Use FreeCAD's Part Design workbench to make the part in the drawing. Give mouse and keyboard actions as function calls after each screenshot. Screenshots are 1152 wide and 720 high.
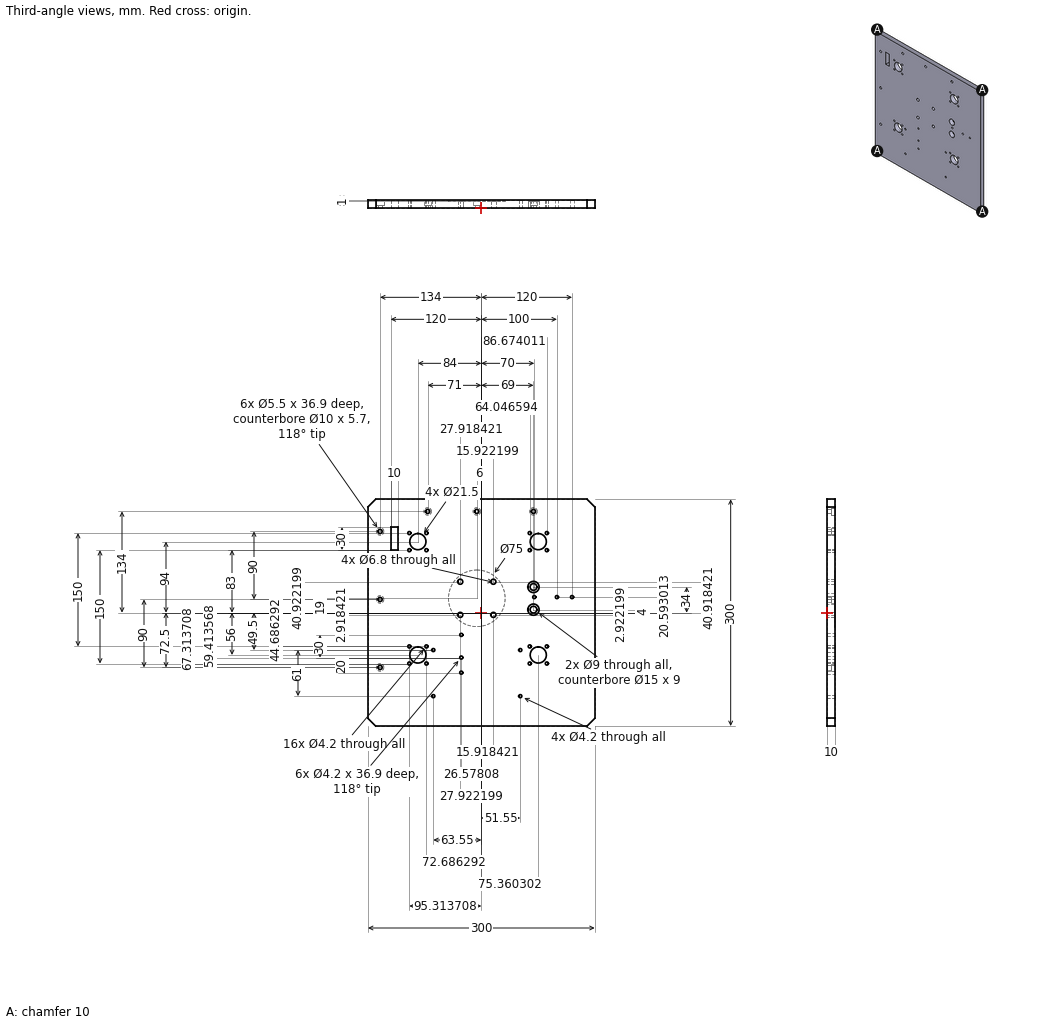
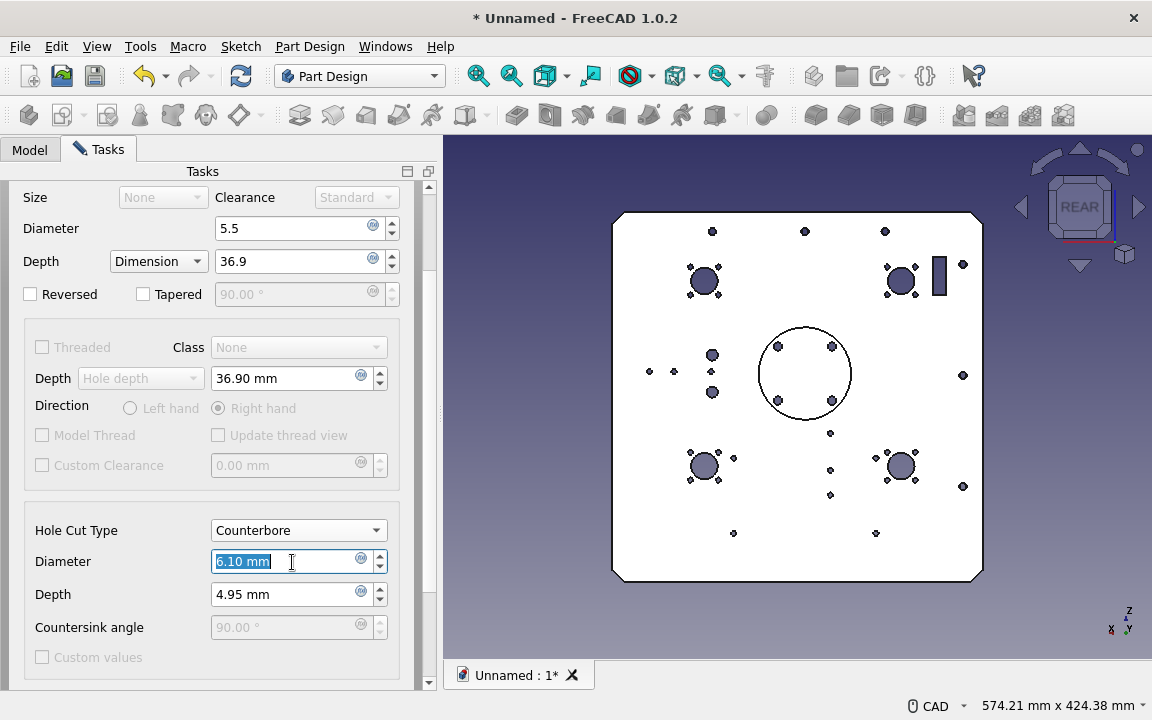
text(10)
key(Tab)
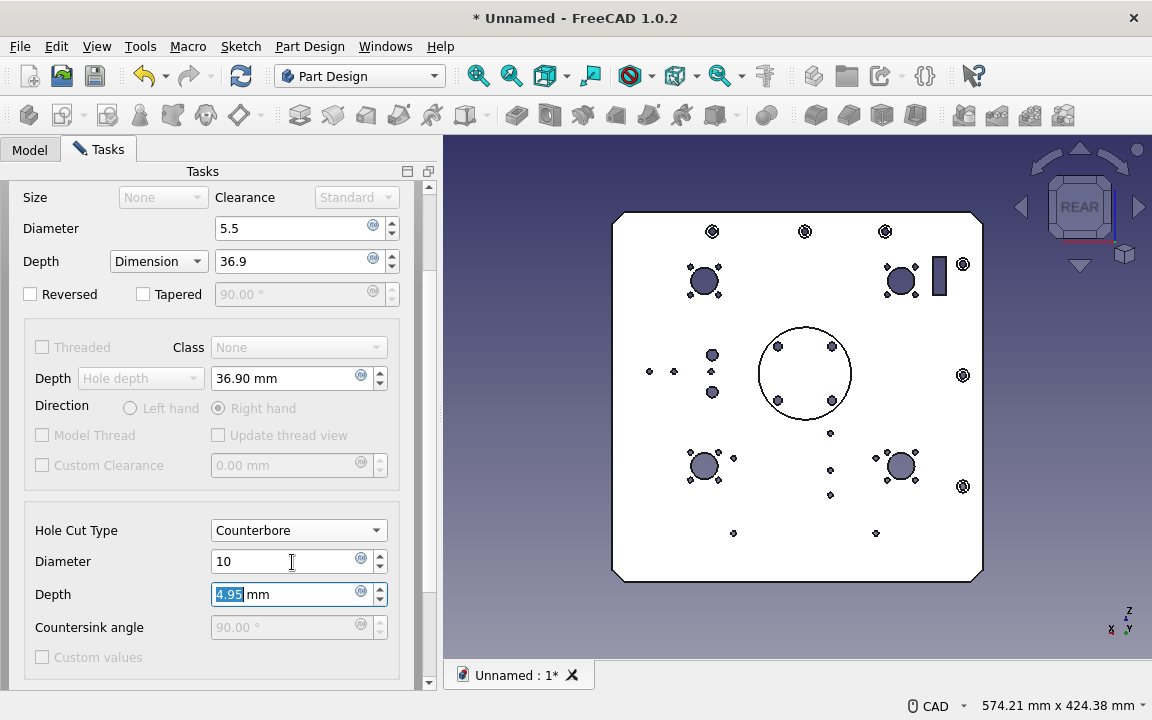
text(5.7)
key(Tab)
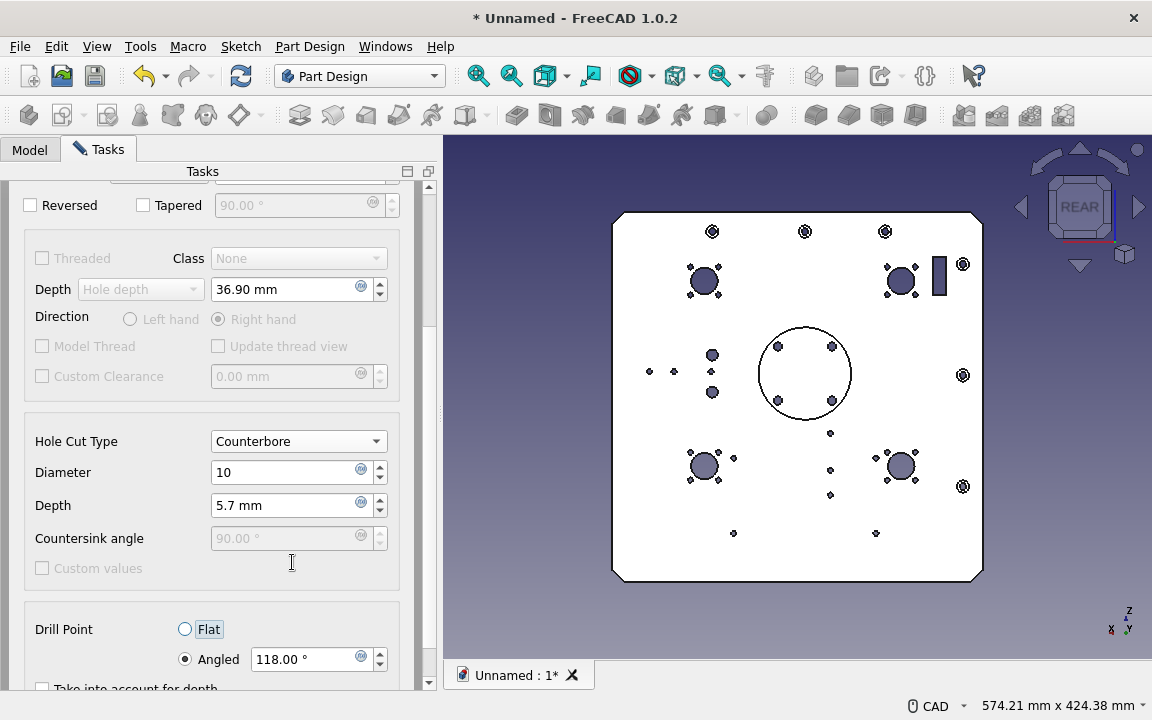
scroll(429, 436, up, 5)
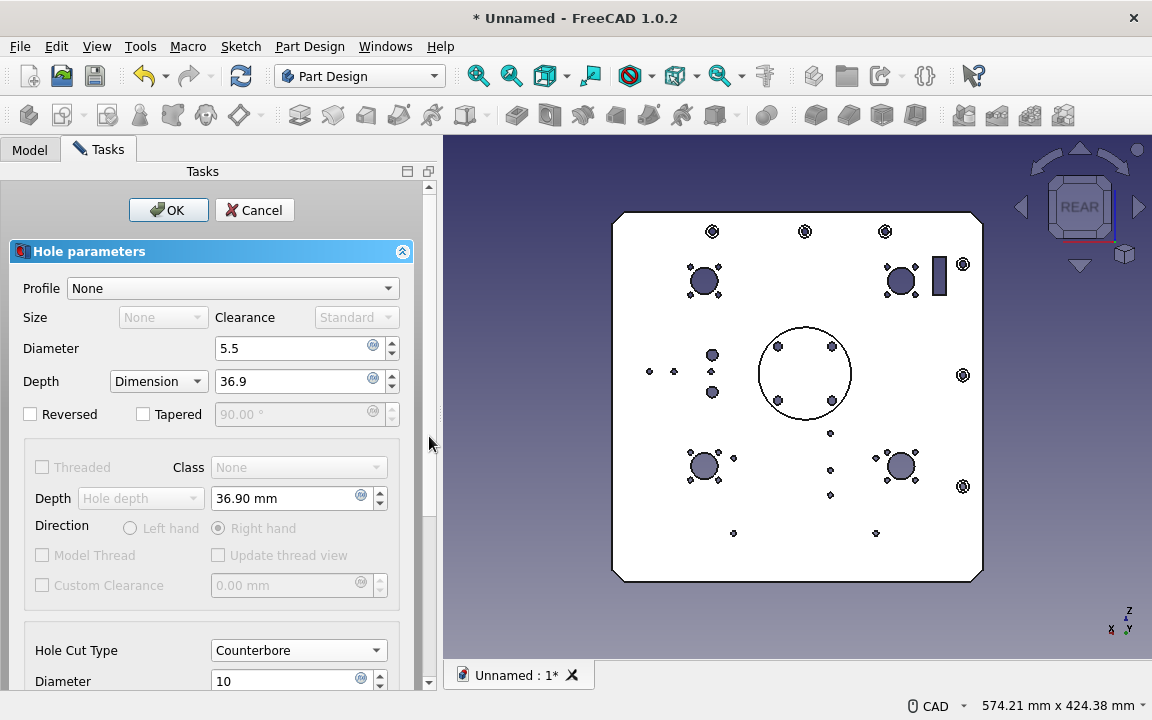
click(169, 210)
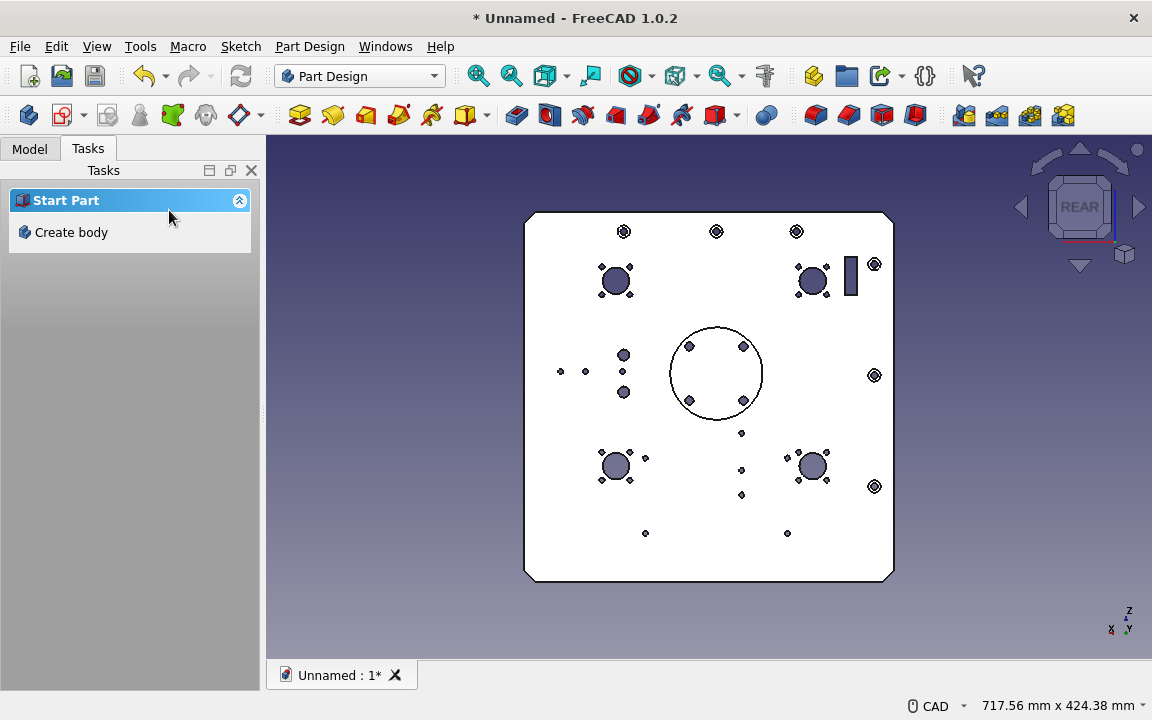
key(0)